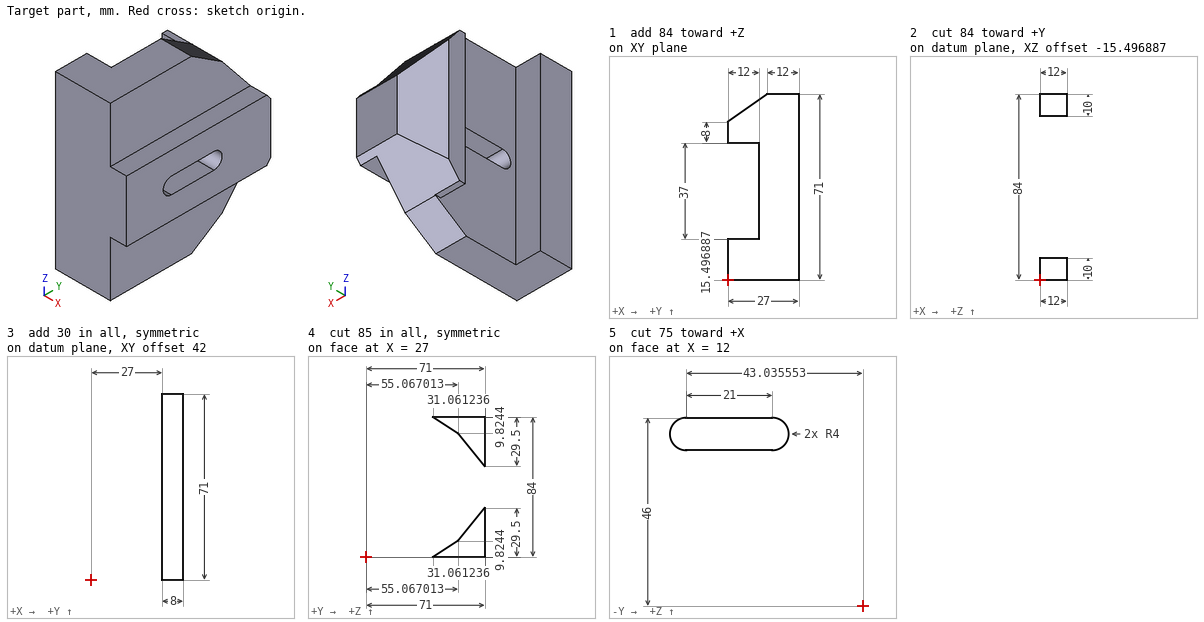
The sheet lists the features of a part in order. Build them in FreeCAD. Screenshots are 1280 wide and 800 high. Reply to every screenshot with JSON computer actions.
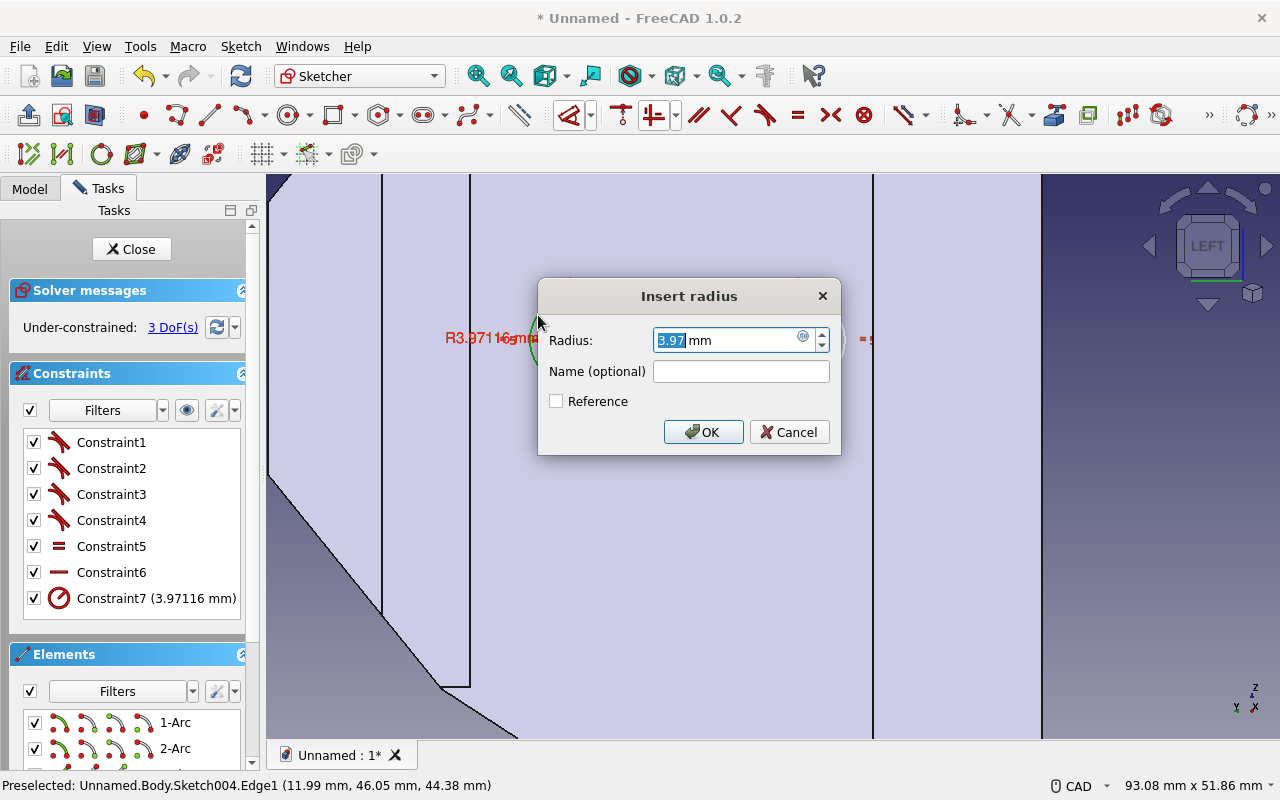
{"action": "type", "text": "4"}
{"action": "key", "text": "Return"}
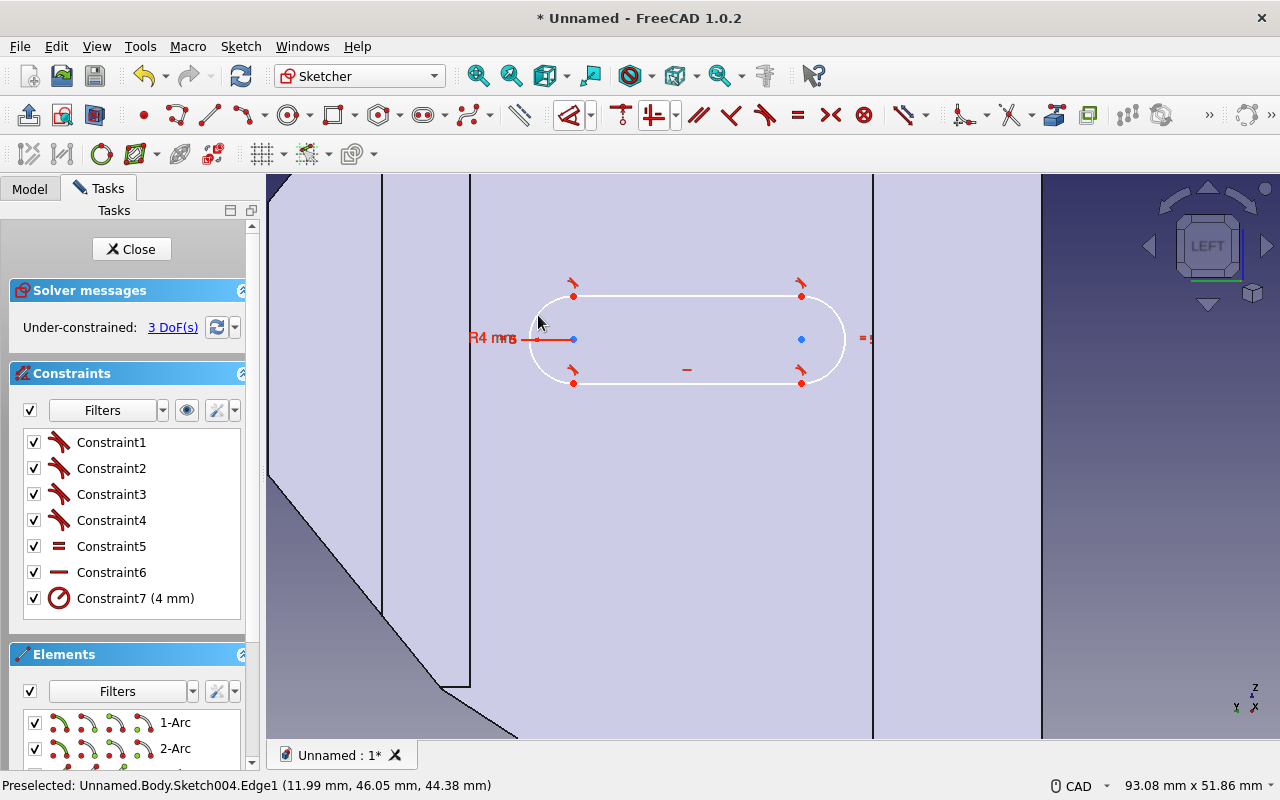
{"action": "left_click", "coordinate": [642, 296]}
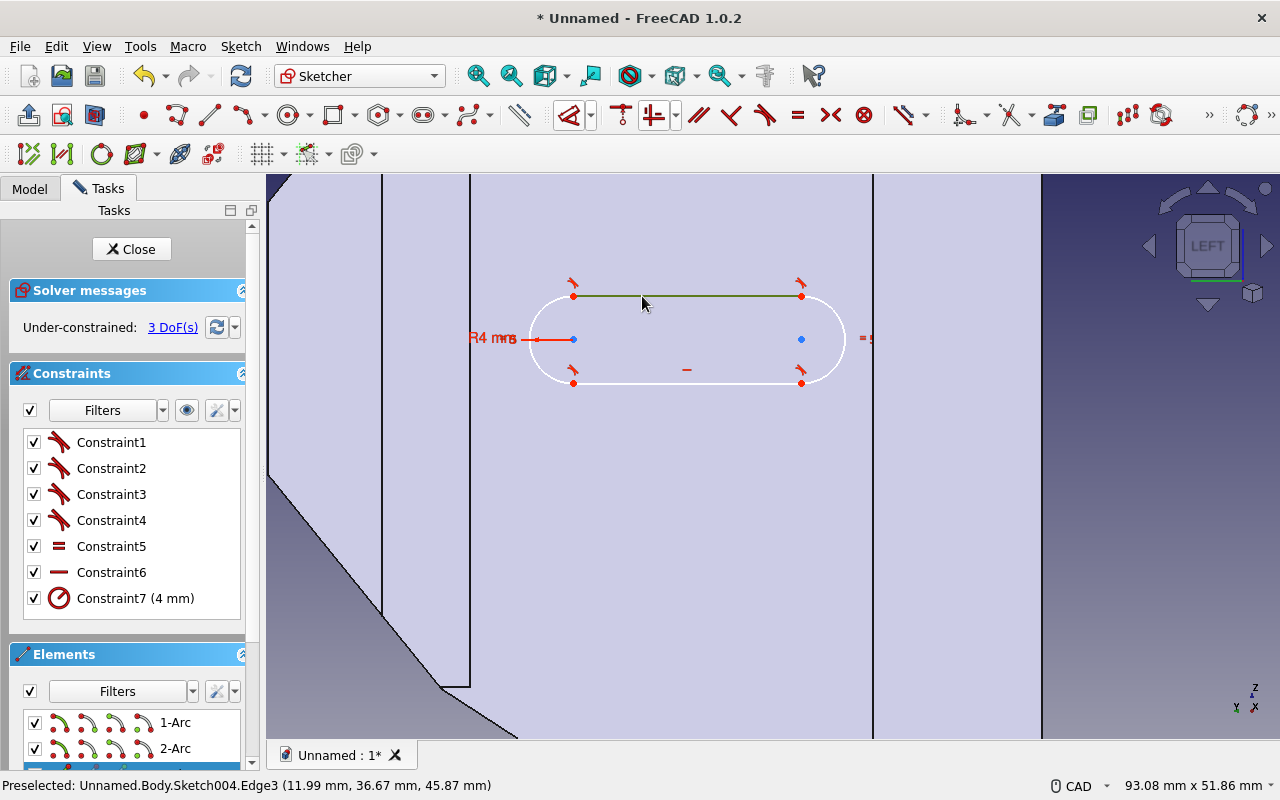
{"action": "key", "text": "l"}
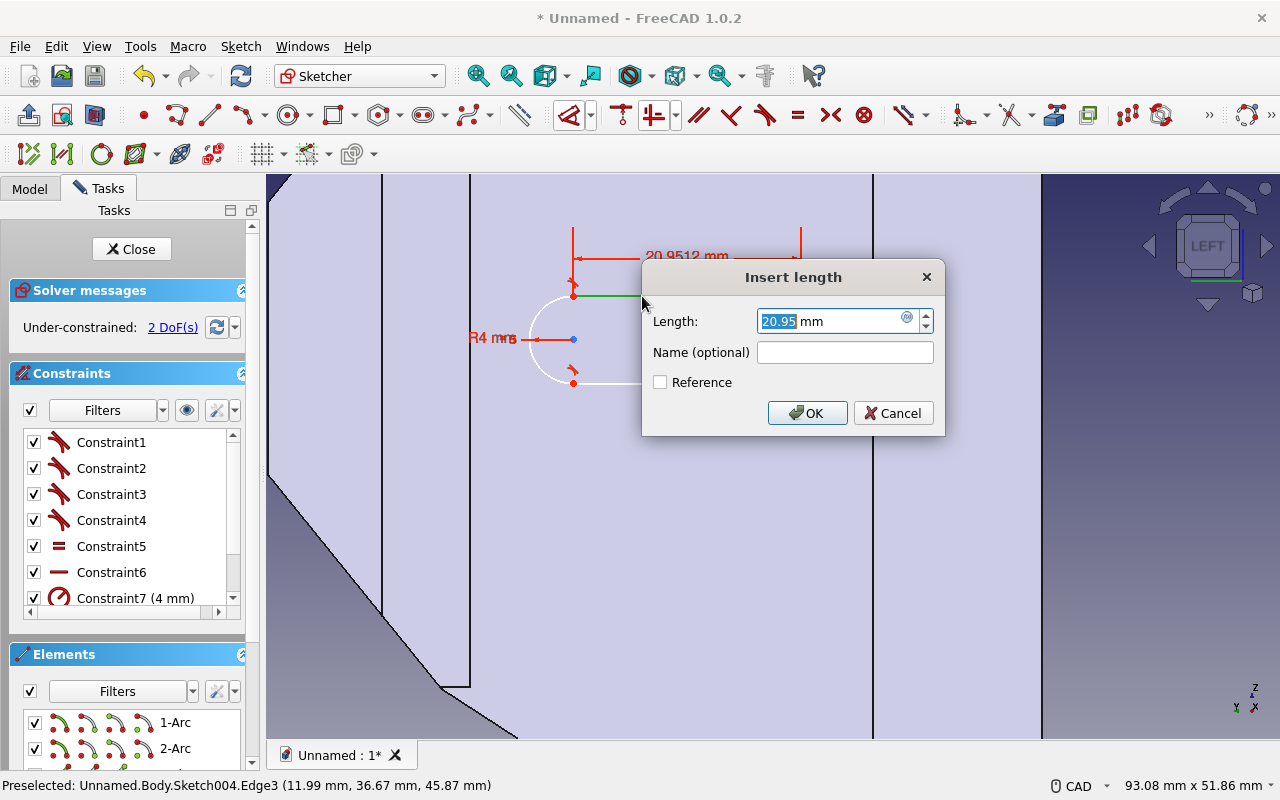
{"action": "type", "text": "21"}
{"action": "key", "text": "Return"}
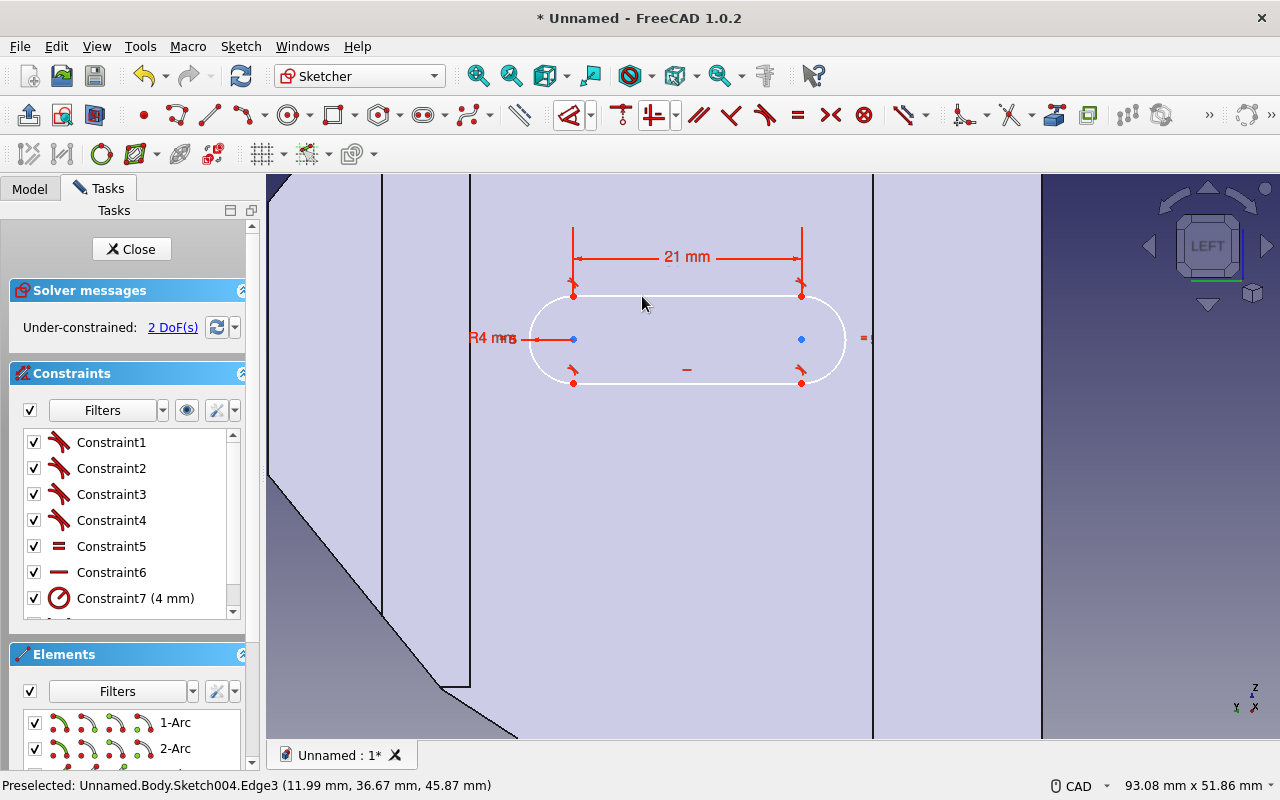
{"action": "left_click", "coordinate": [573, 296]}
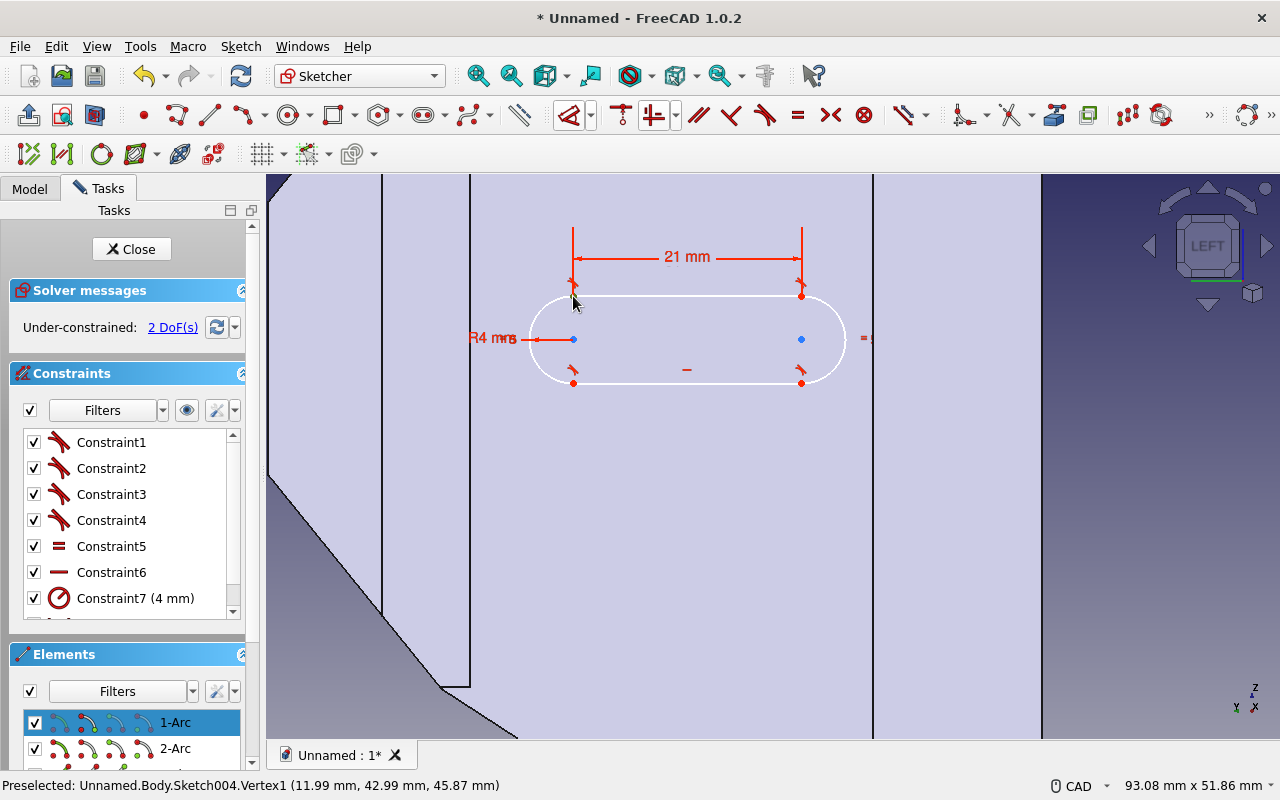
{"action": "left_click", "coordinate": [590, 116]}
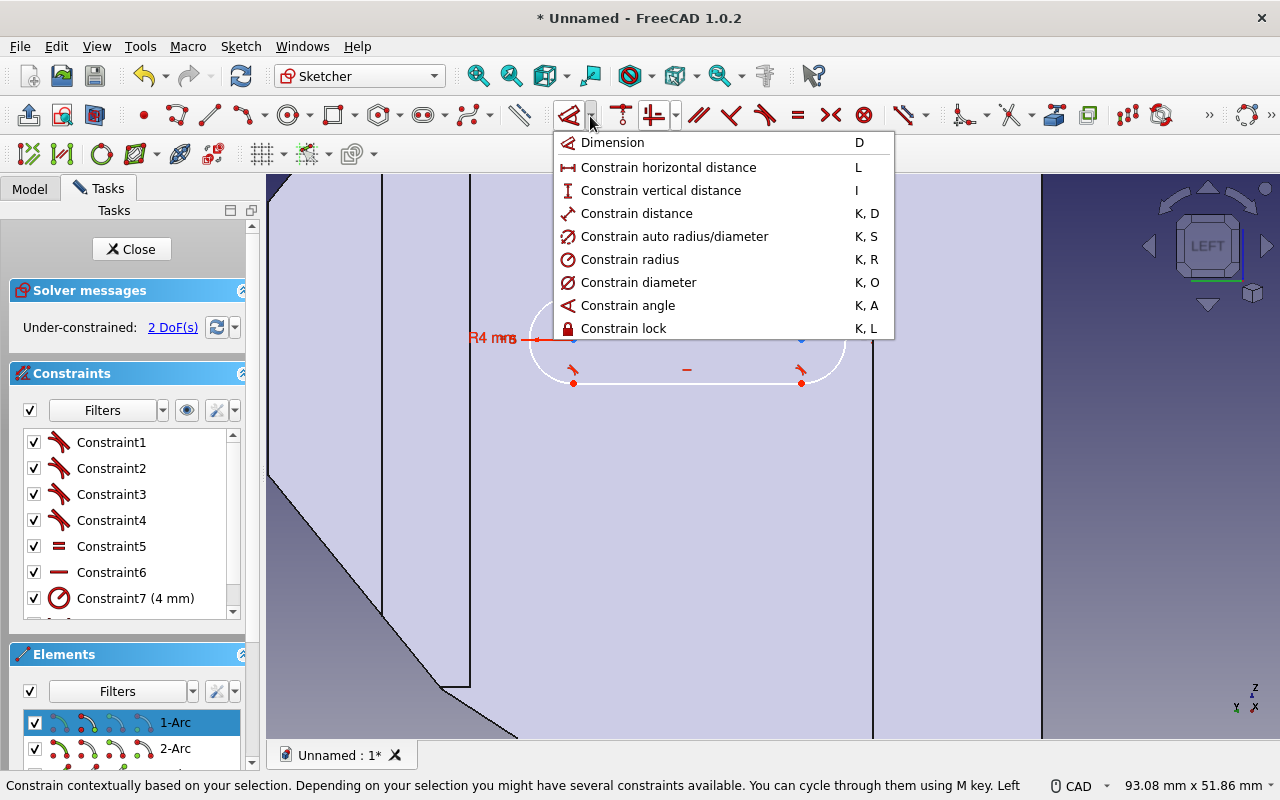
{"action": "left_click", "coordinate": [724, 190]}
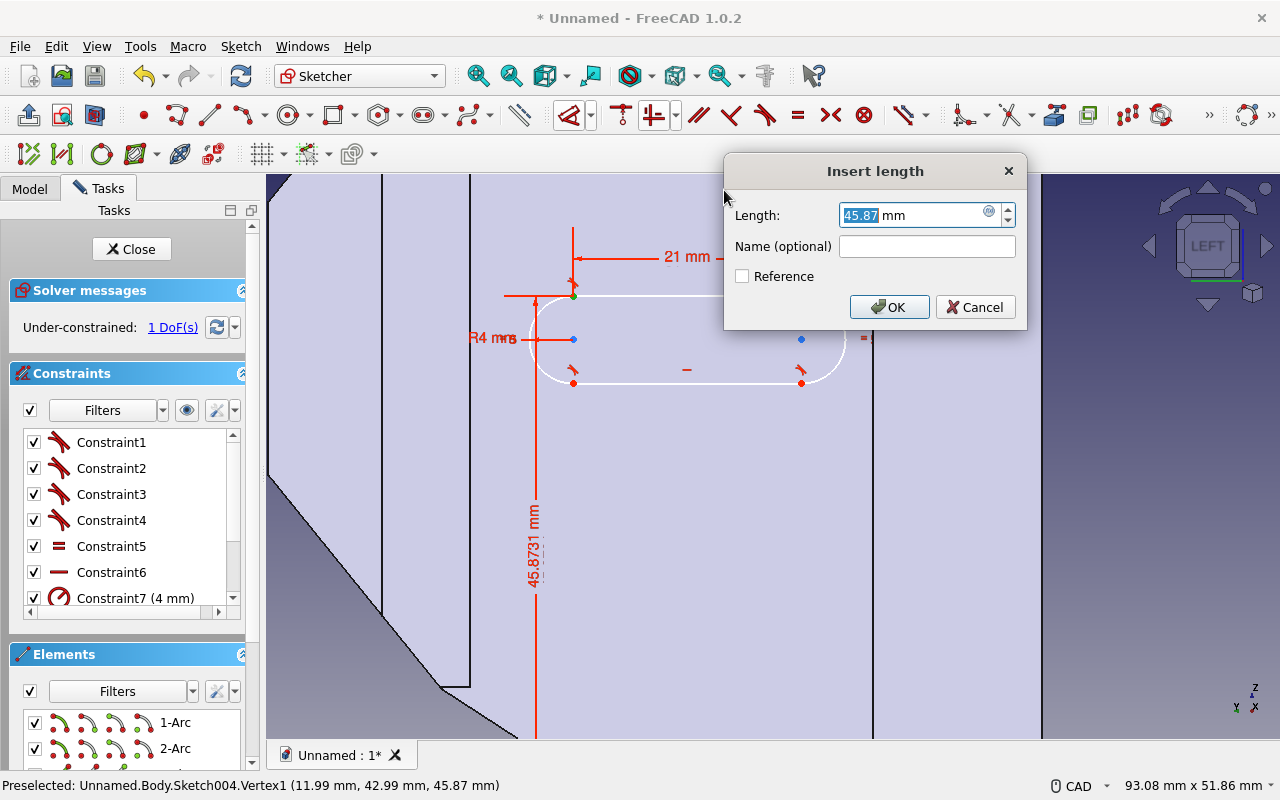
{"action": "type", "text": "46"}
{"action": "key", "text": "Return"}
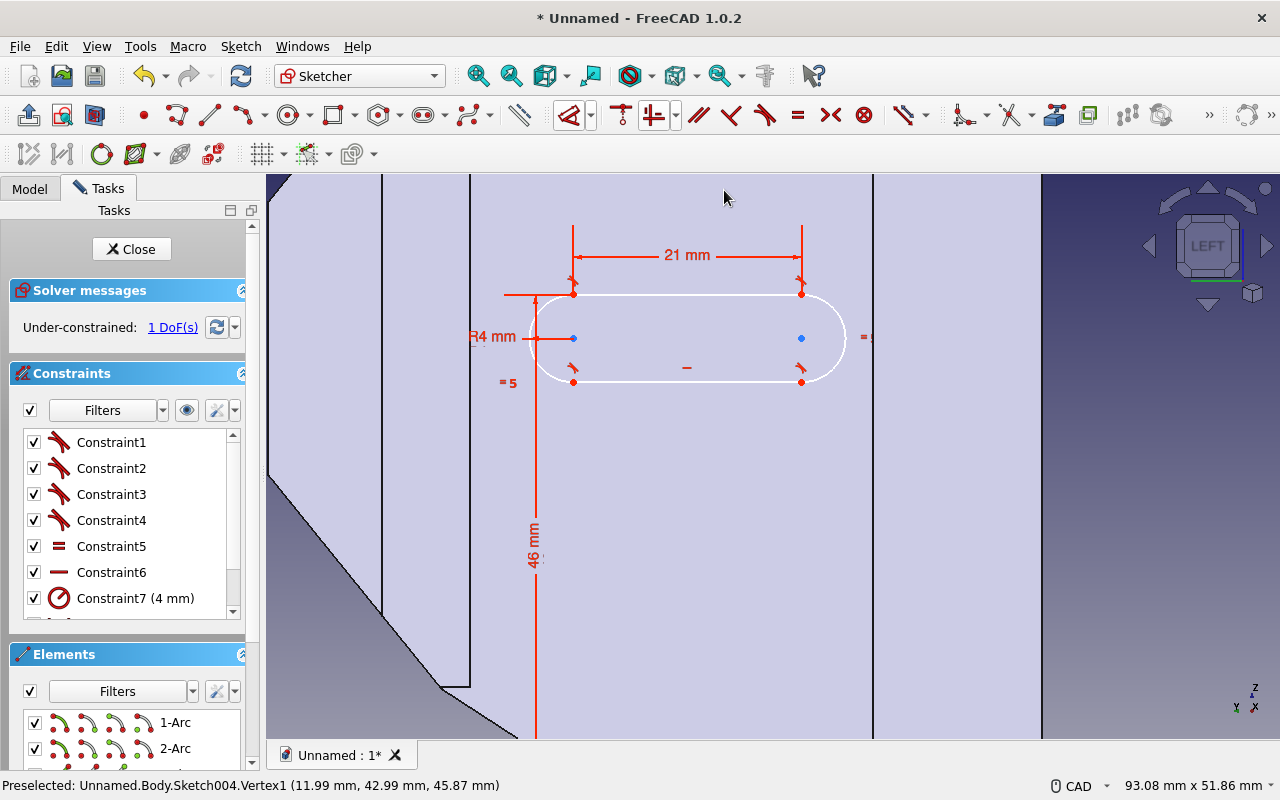
{"action": "left_click", "coordinate": [573, 295]}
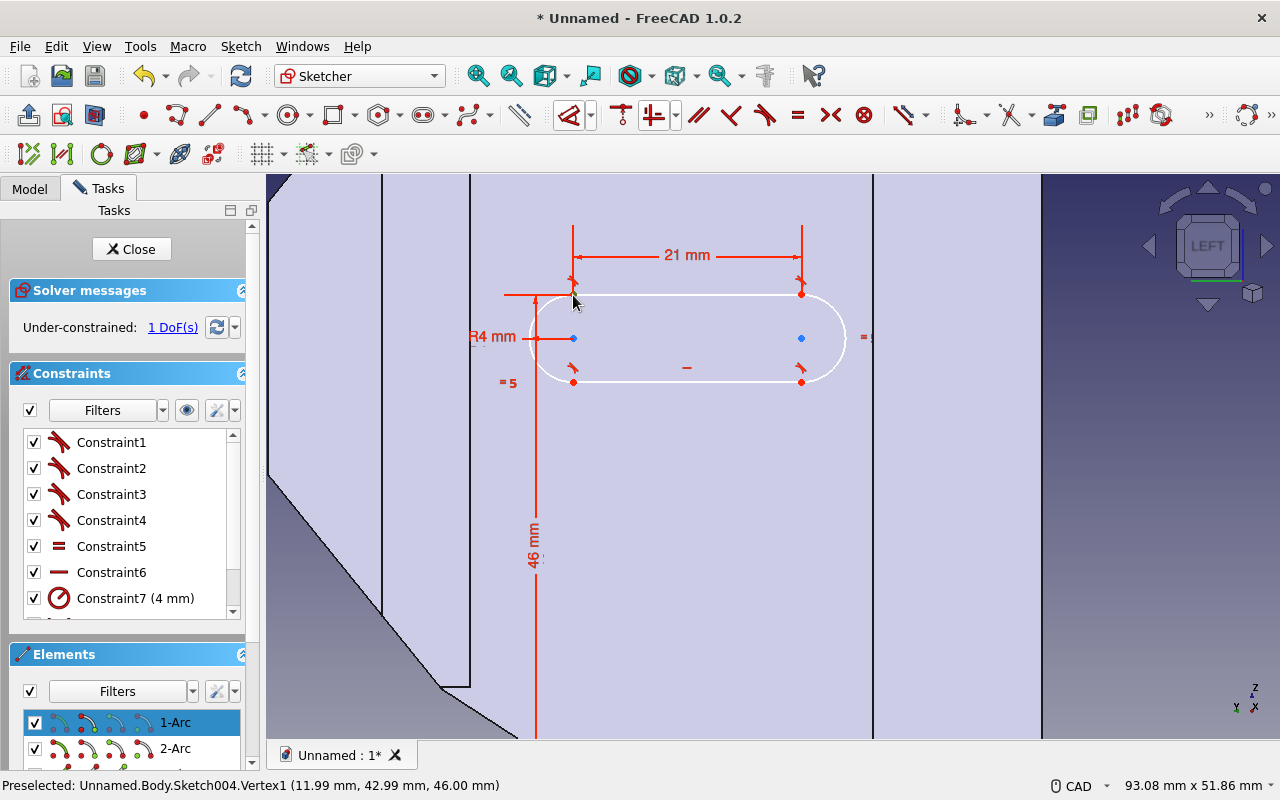
{"action": "left_click", "coordinate": [590, 116]}